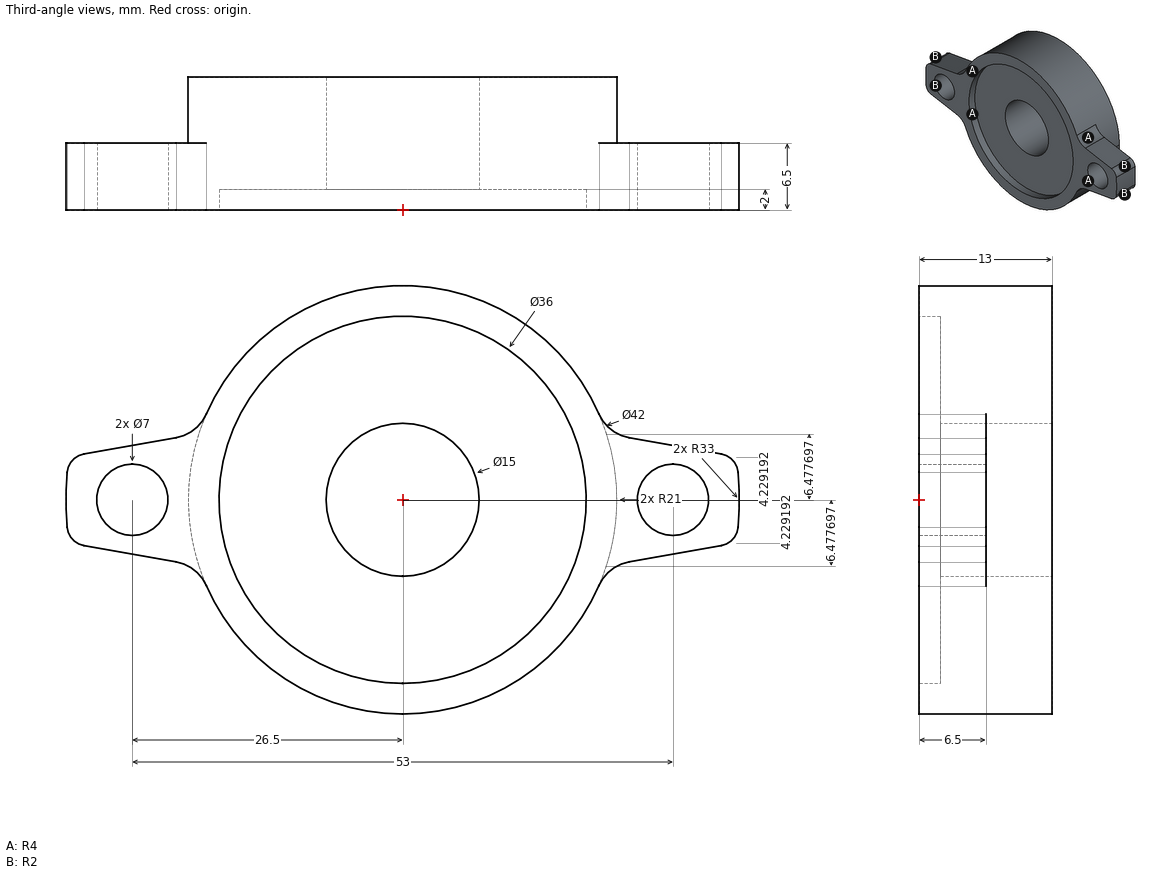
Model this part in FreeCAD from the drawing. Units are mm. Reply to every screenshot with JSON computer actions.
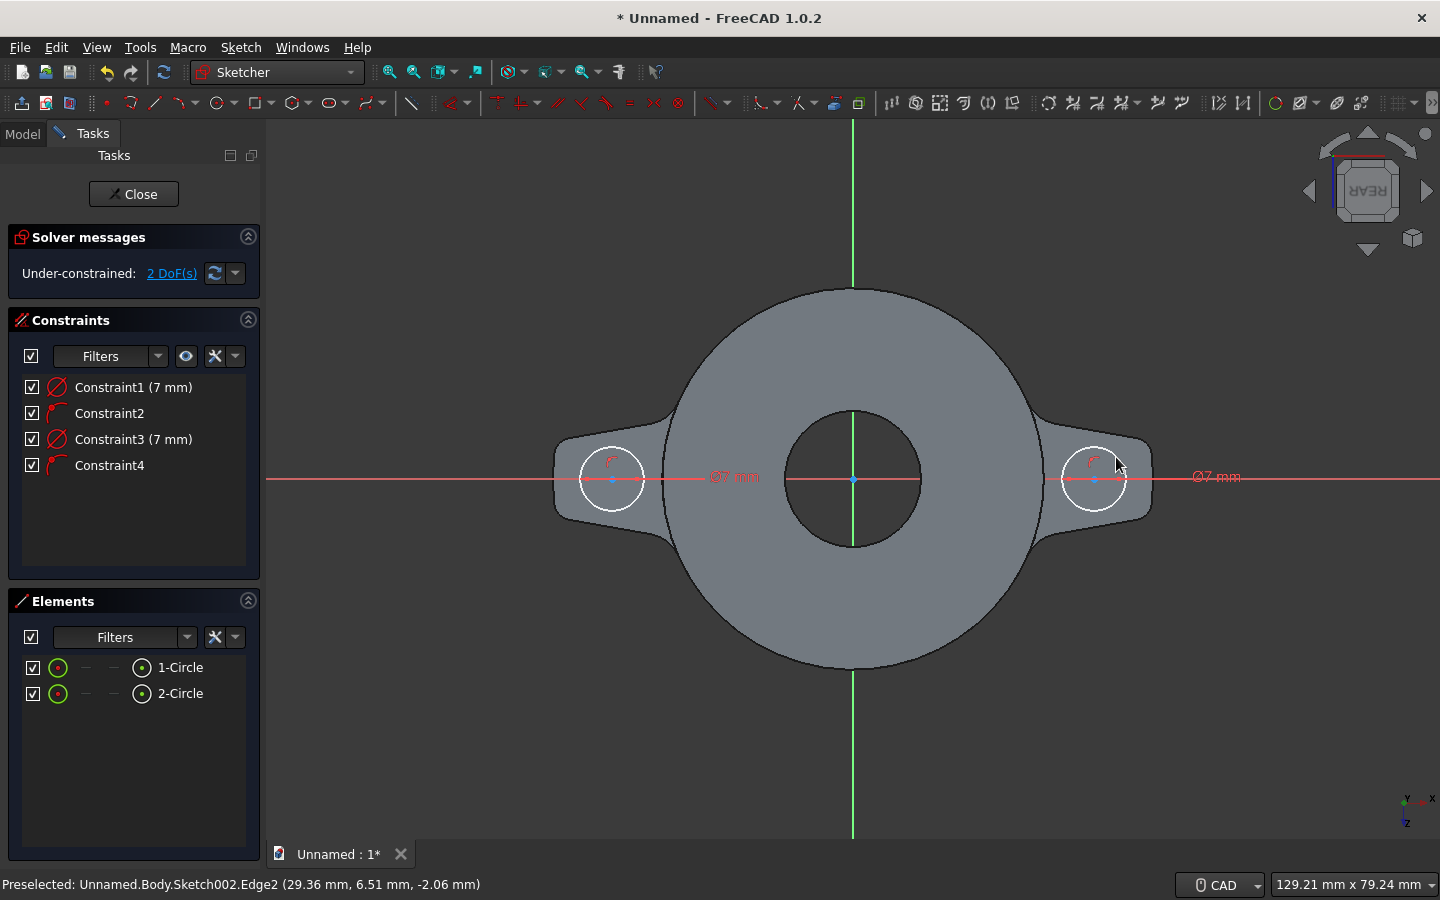
{"action": "left_click", "coordinate": [450, 104]}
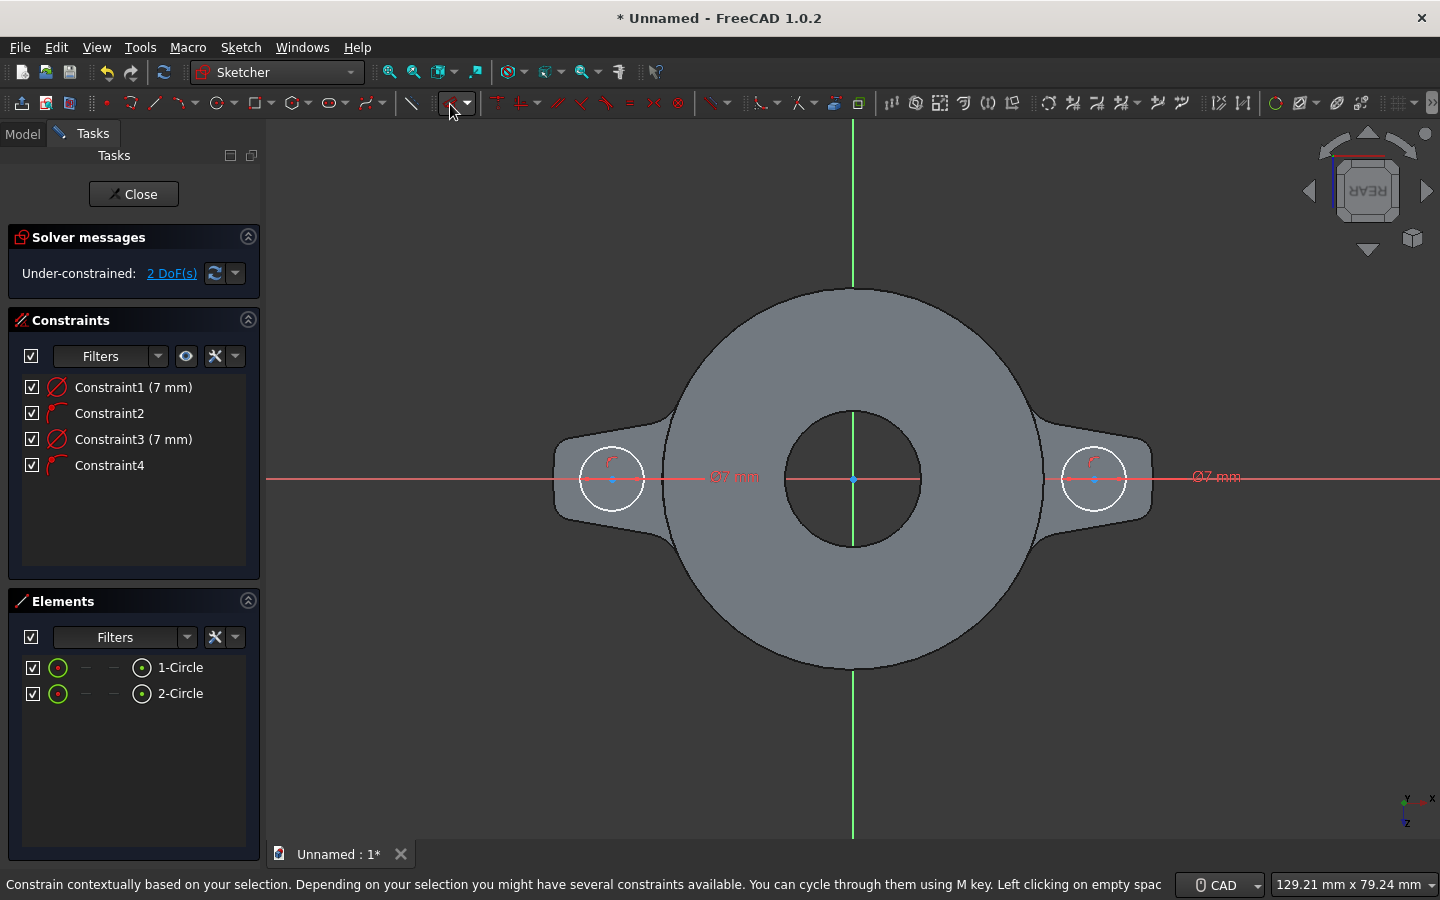
{"action": "left_click", "coordinate": [612, 479]}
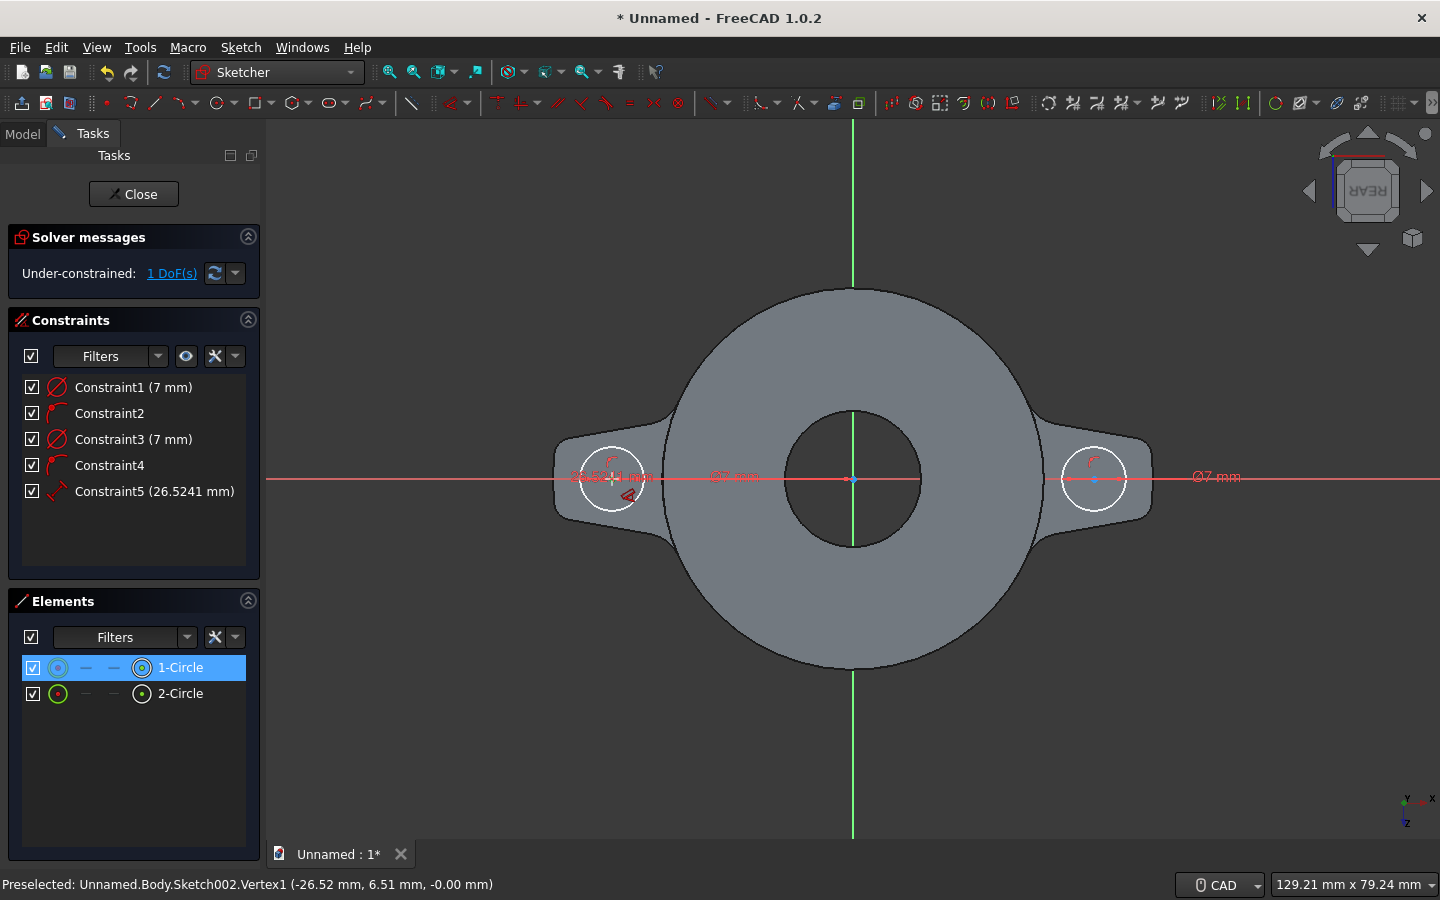
{"action": "left_click", "coordinate": [1094, 479]}
{"action": "left_click", "coordinate": [742, 513]}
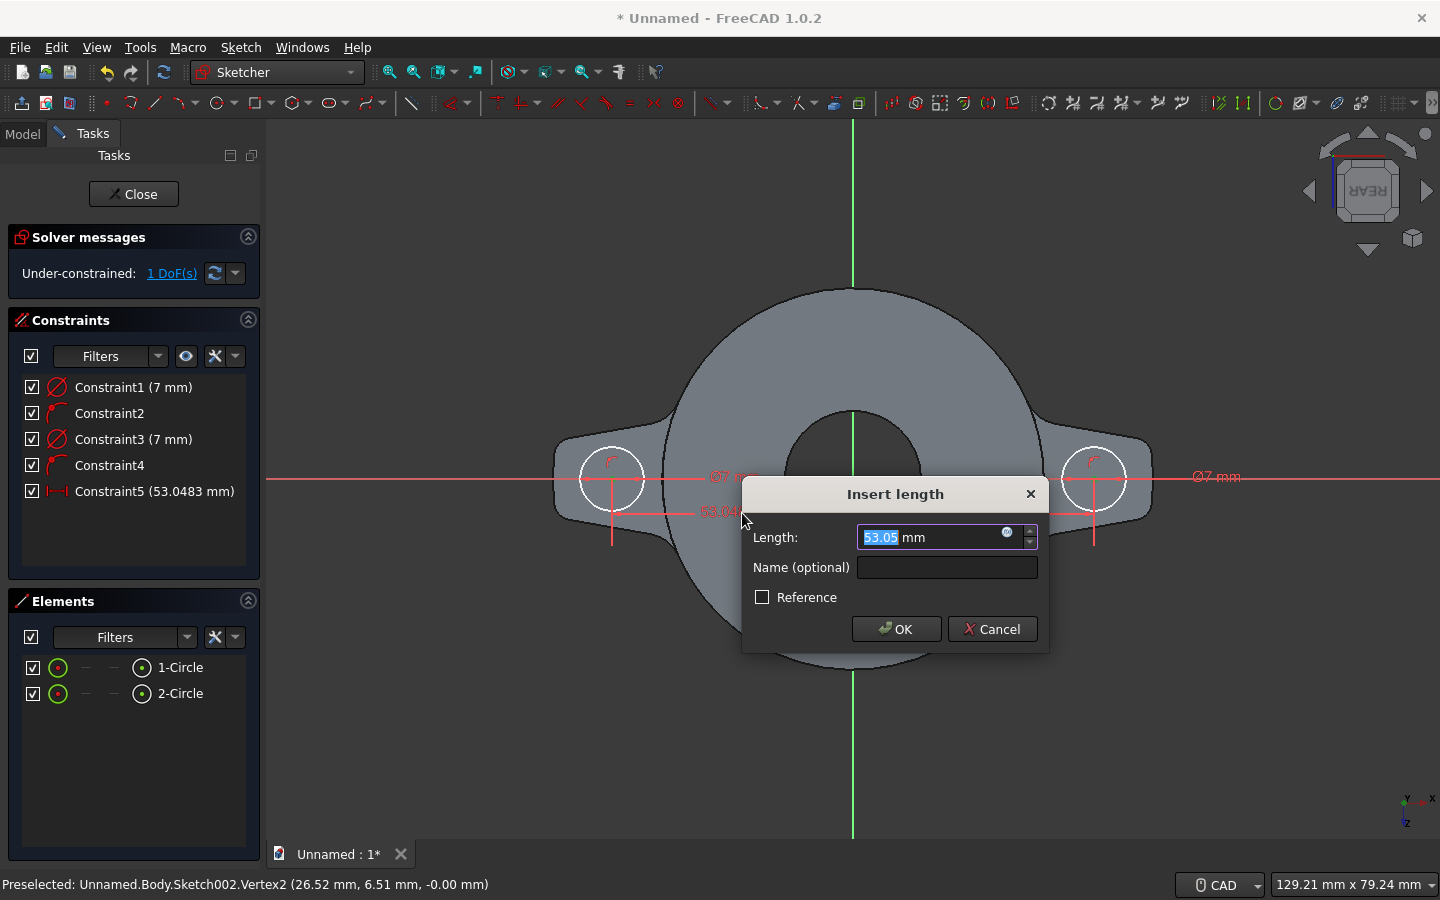
{"action": "type", "text": "53"}
{"action": "key", "text": "Return"}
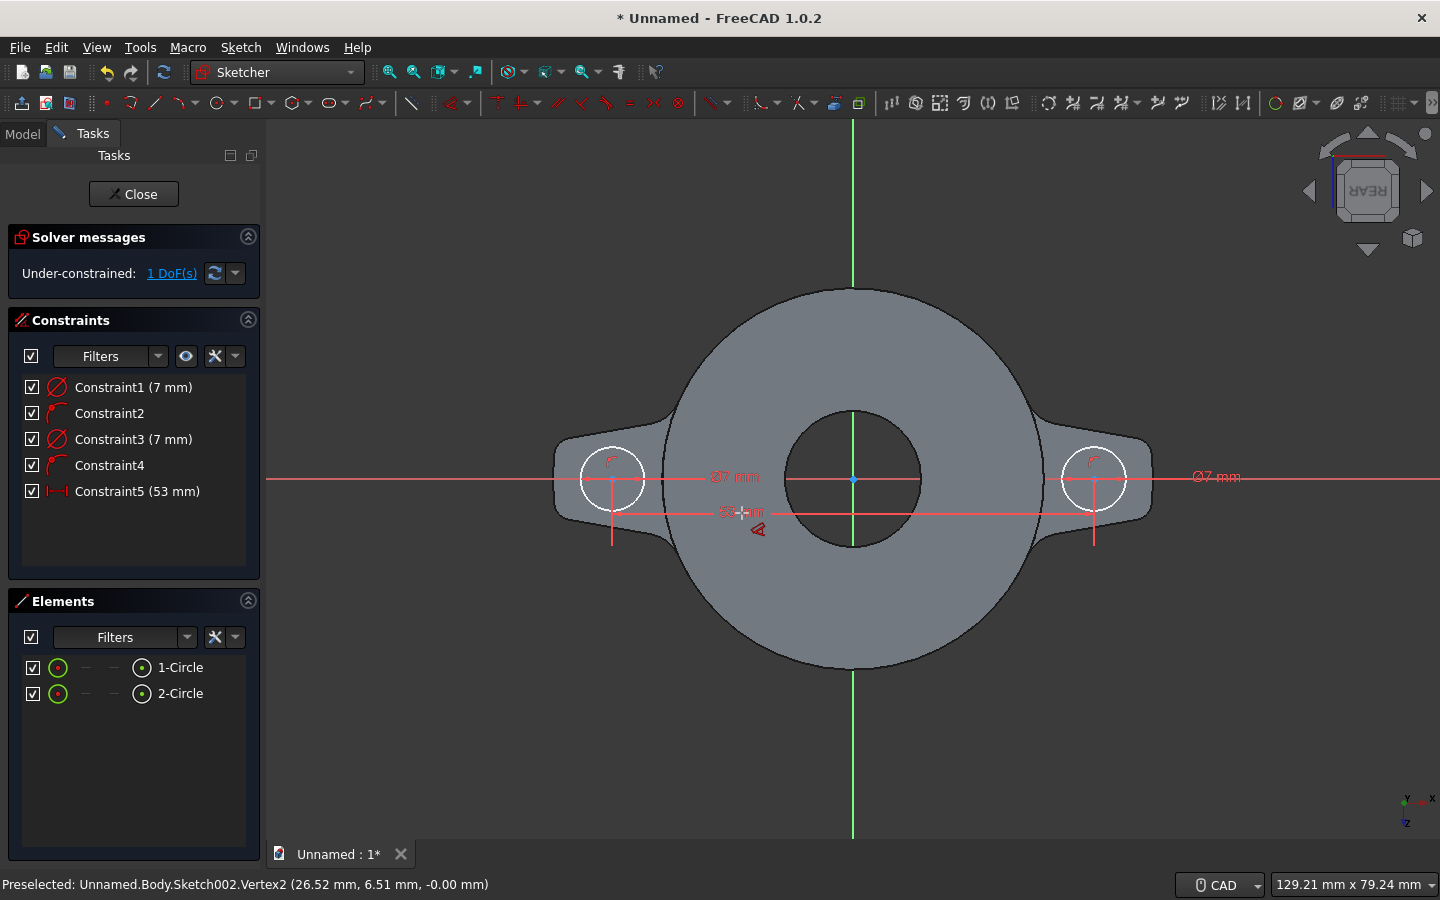
{"action": "left_click", "coordinate": [612, 479]}
{"action": "left_click", "coordinate": [649, 513]}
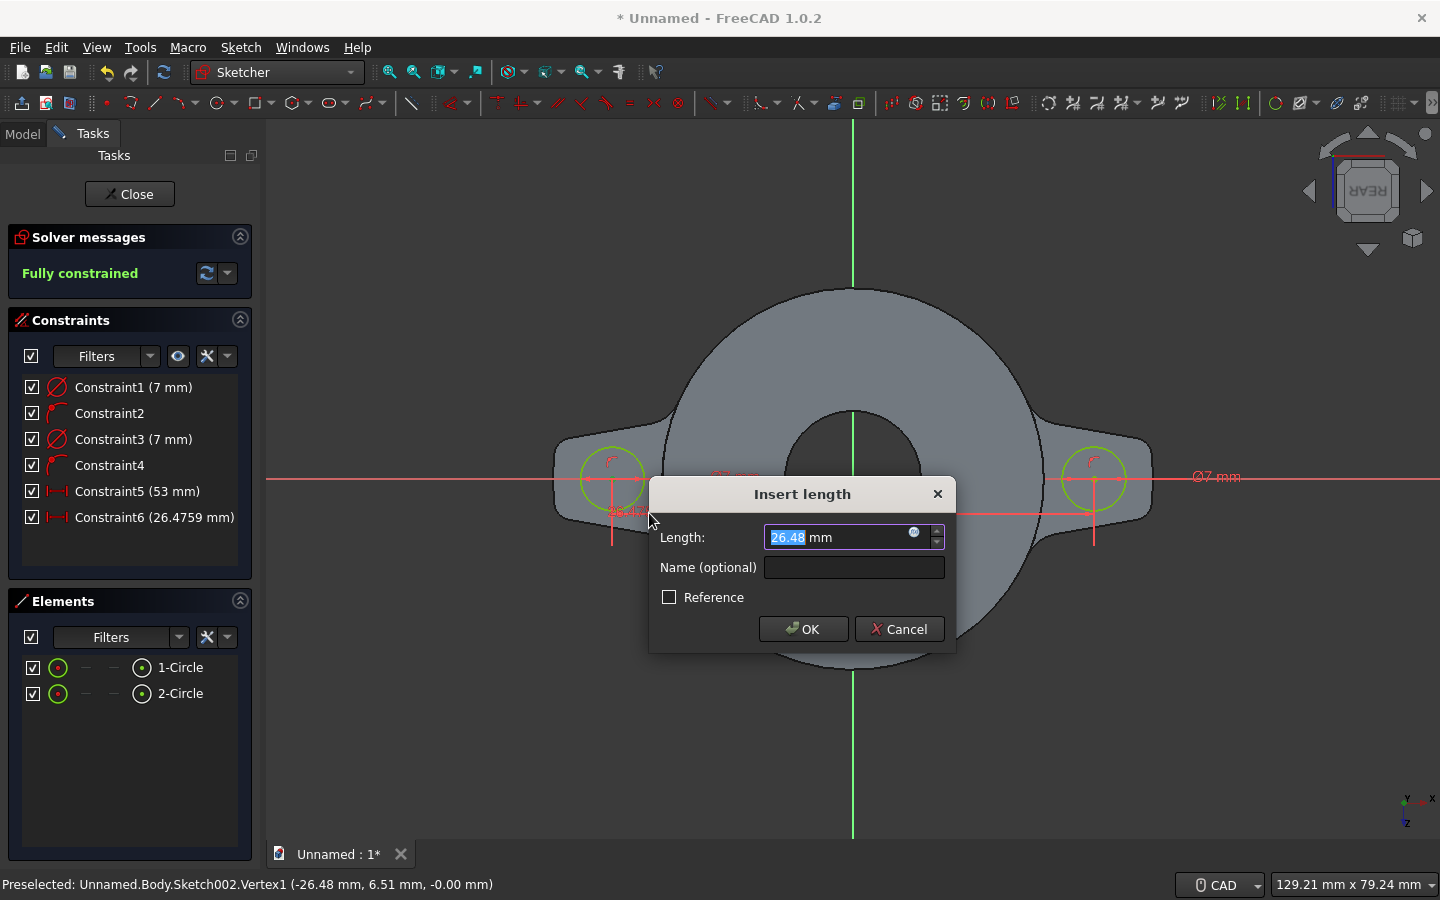
{"action": "type", "text": "26.5"}
{"action": "key", "text": "Return"}
{"action": "key", "text": "Escape"}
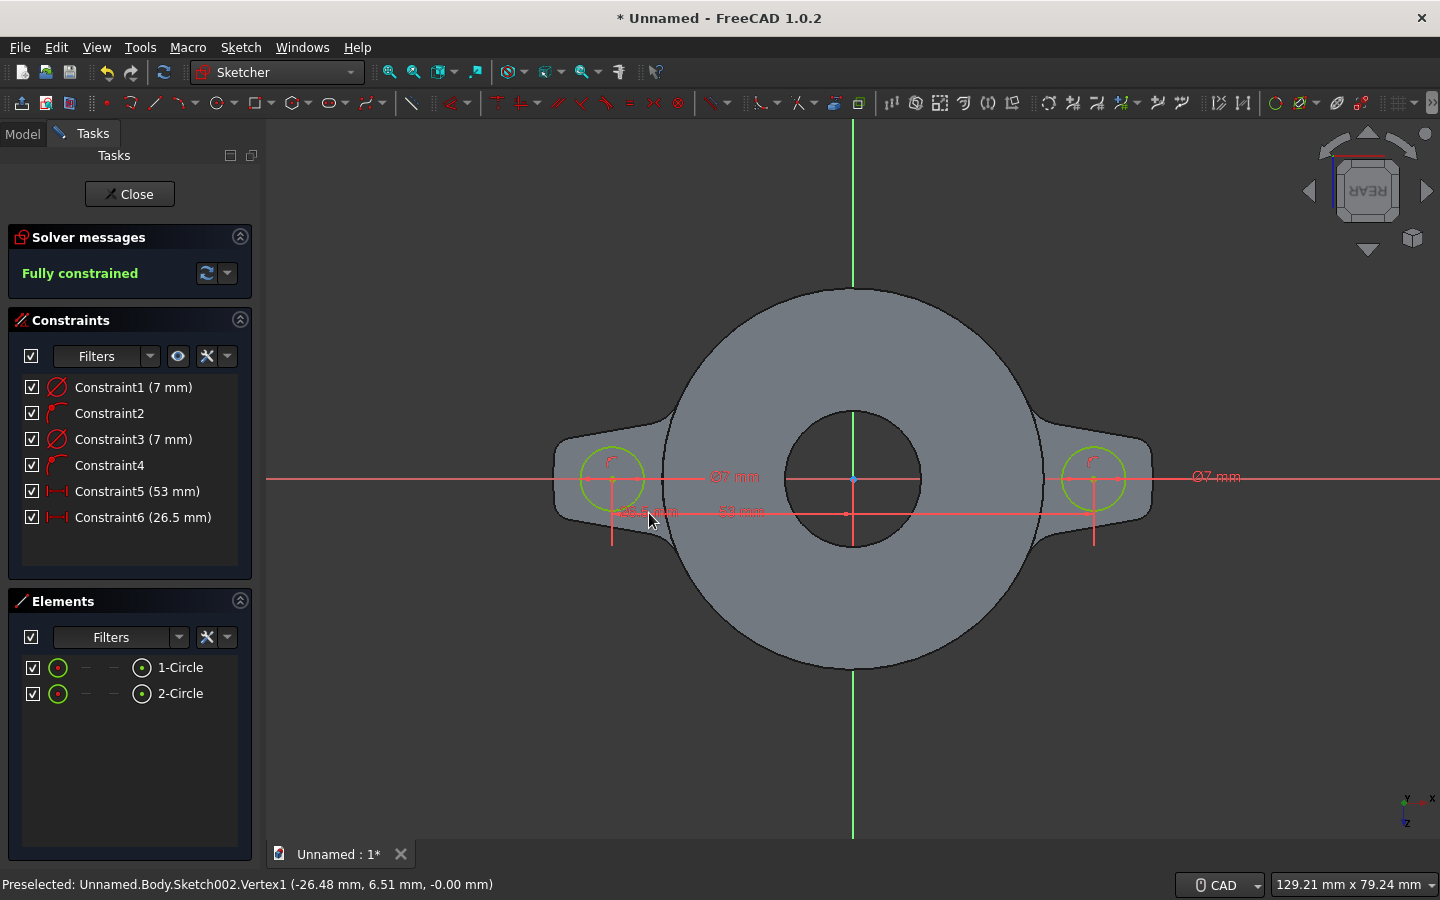
{"action": "left_click", "coordinate": [130, 194]}